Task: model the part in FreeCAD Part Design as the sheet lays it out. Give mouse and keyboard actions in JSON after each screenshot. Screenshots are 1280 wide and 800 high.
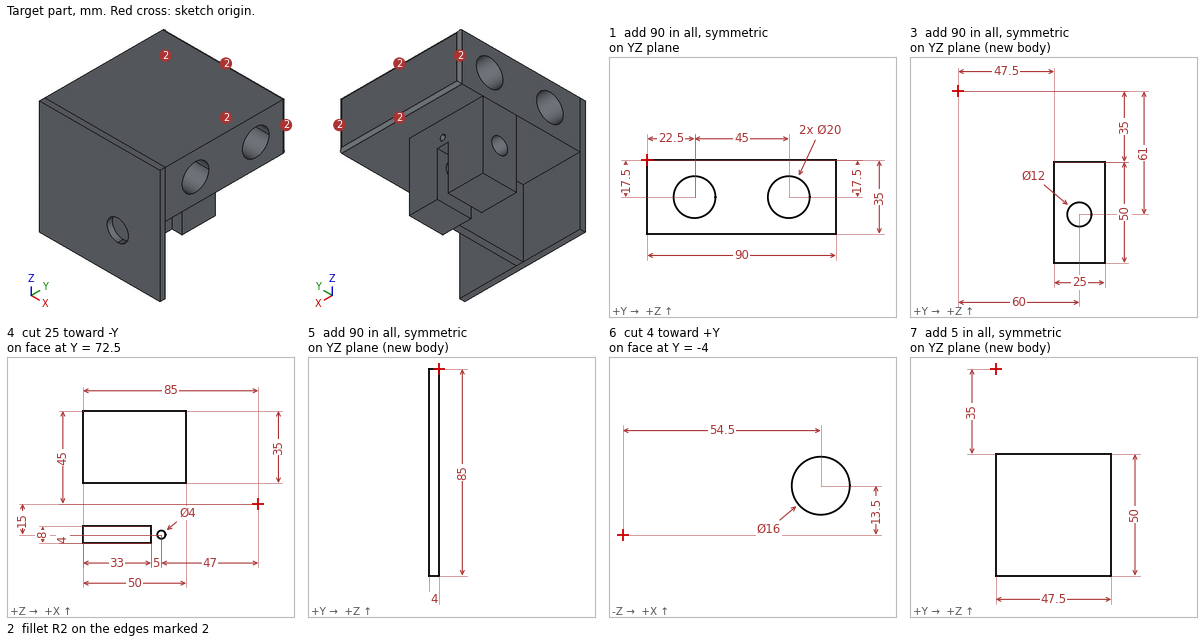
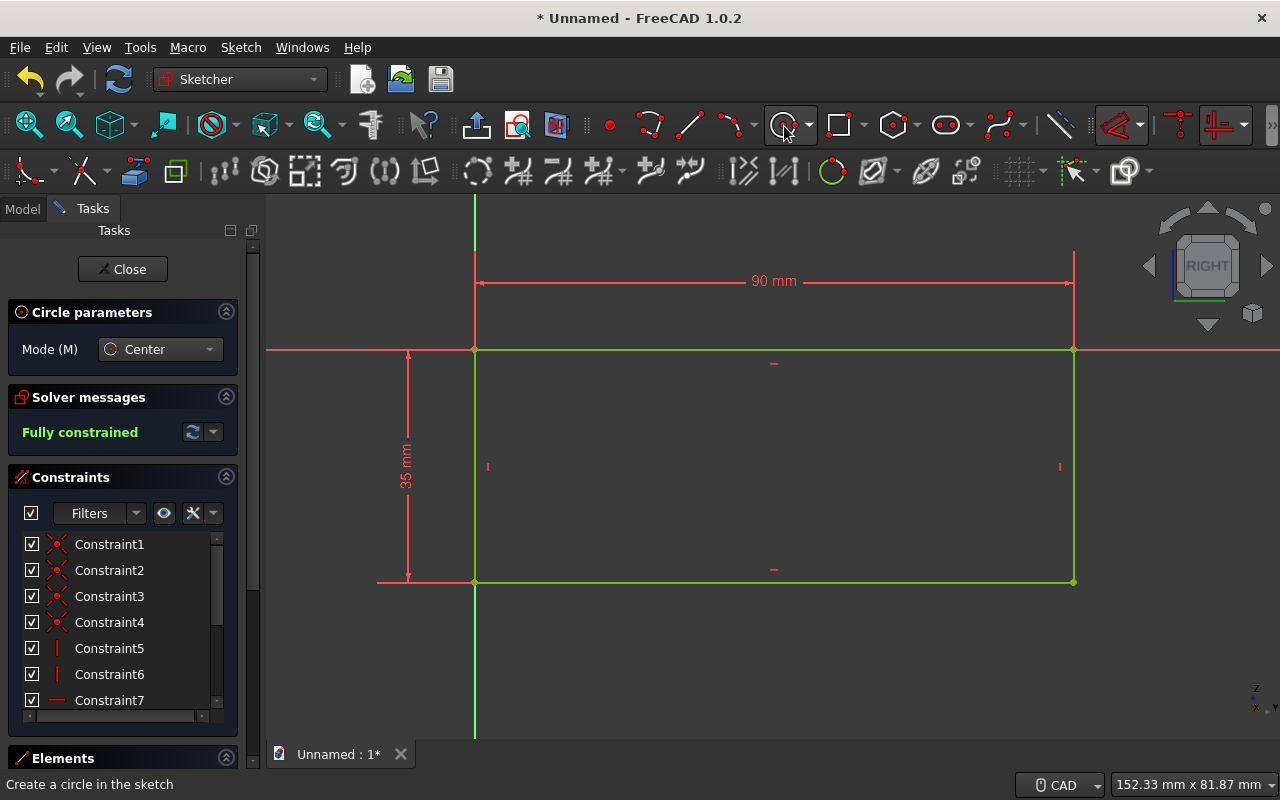
{"action": "left_click", "coordinate": [625, 466]}
{"action": "mouse_move", "coordinate": [672, 419]}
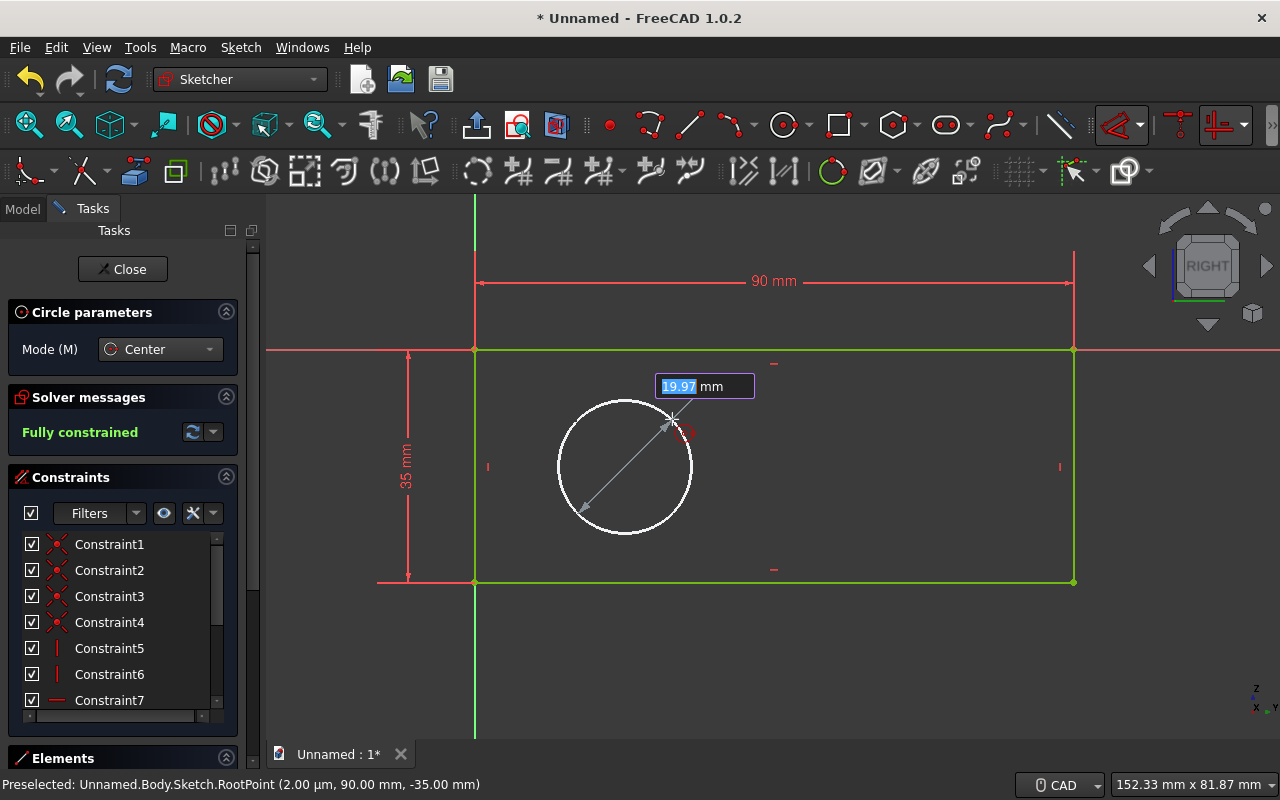
{"action": "type", "text": "20"}
{"action": "key", "text": "Return"}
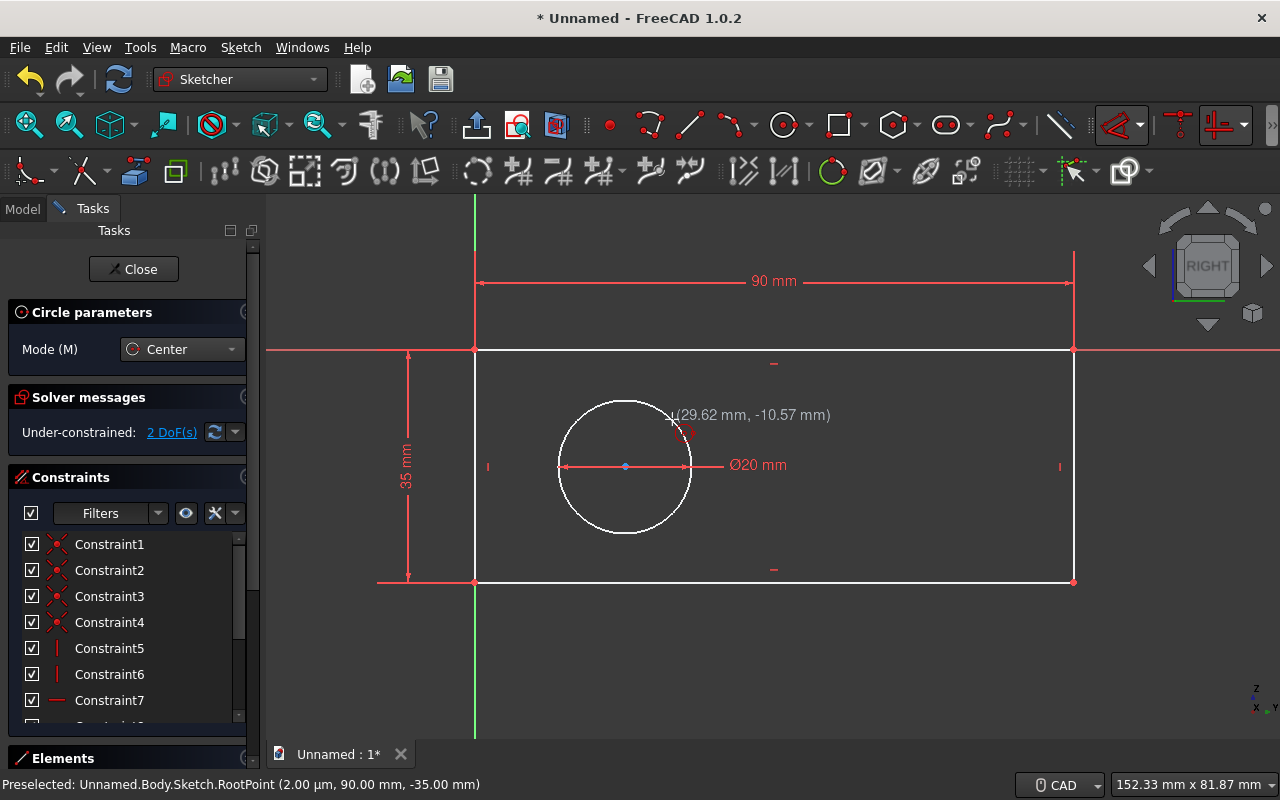
{"action": "left_click", "coordinate": [924, 466]}
{"action": "mouse_move", "coordinate": [971, 419]}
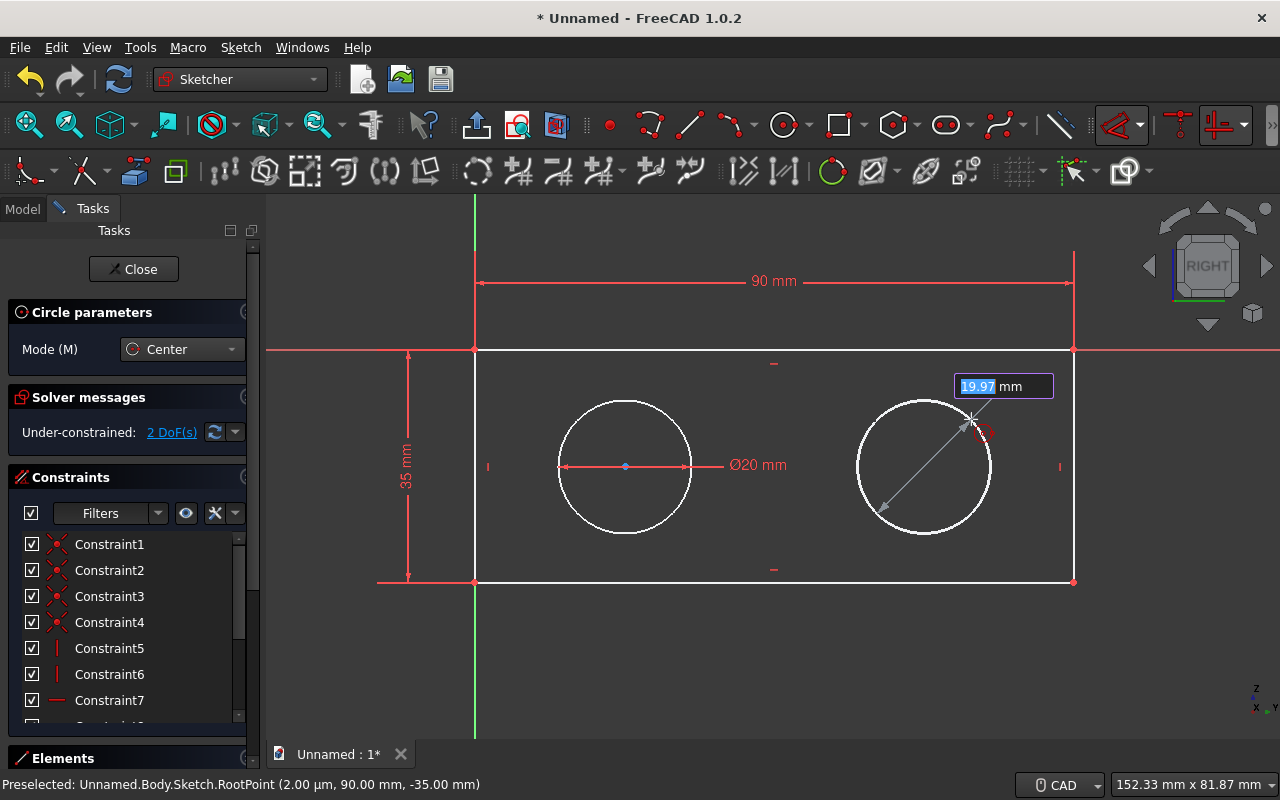
{"action": "type", "text": "20"}
{"action": "key", "text": "Return"}
{"action": "key", "text": "Escape"}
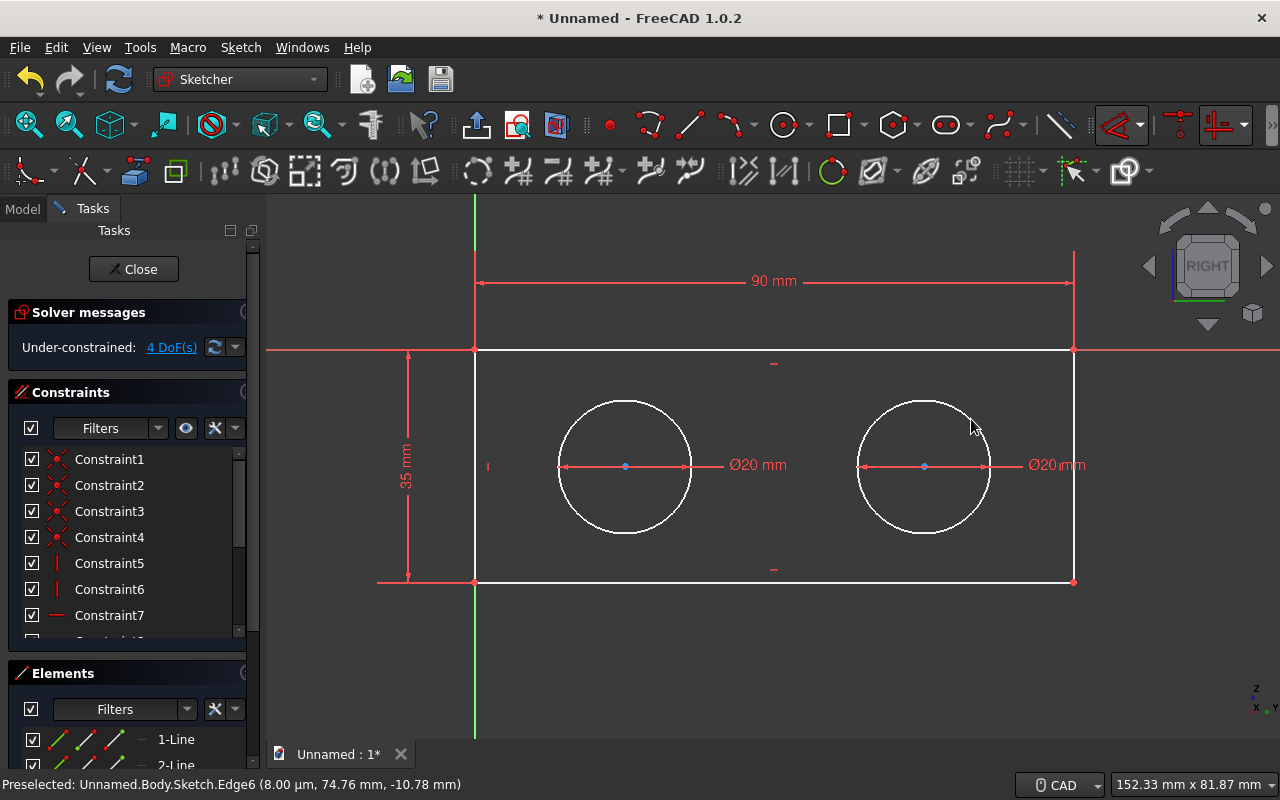
{"action": "left_click", "coordinate": [1116, 126]}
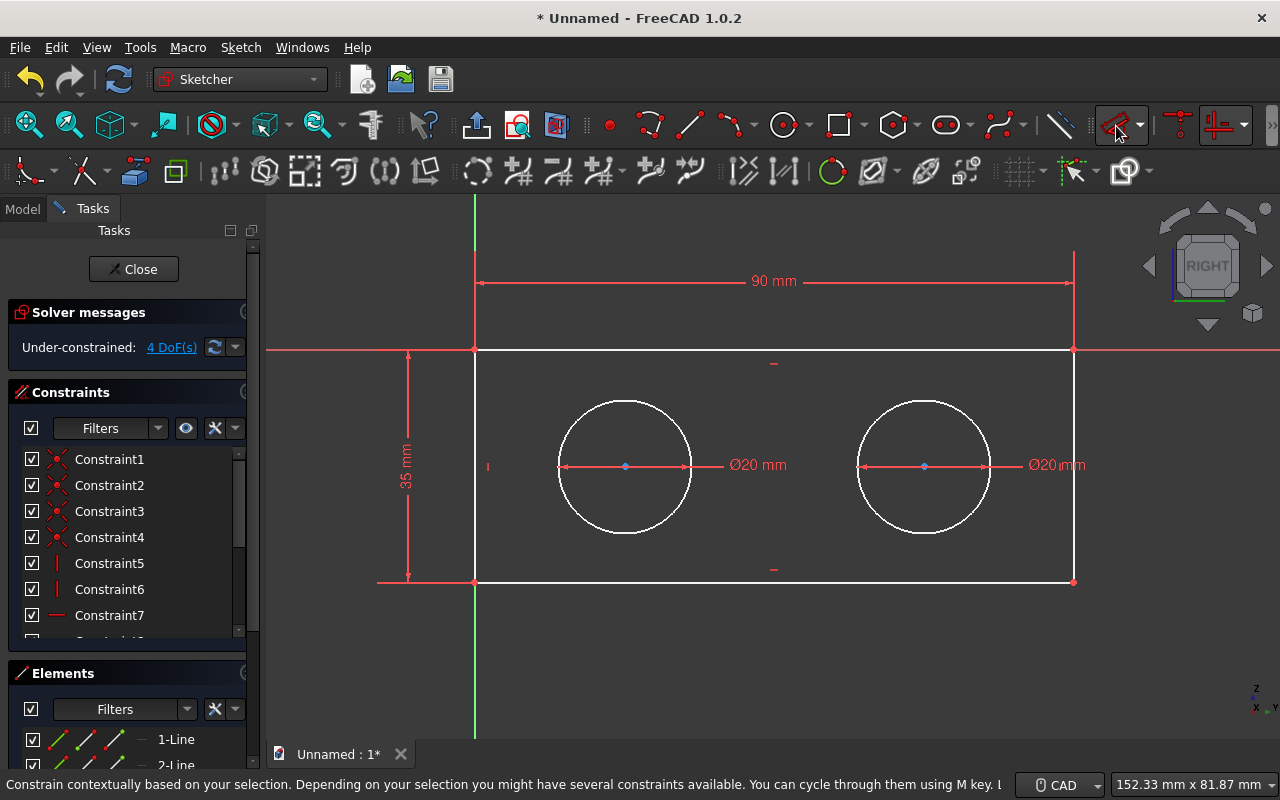
{"action": "left_click", "coordinate": [625, 467]}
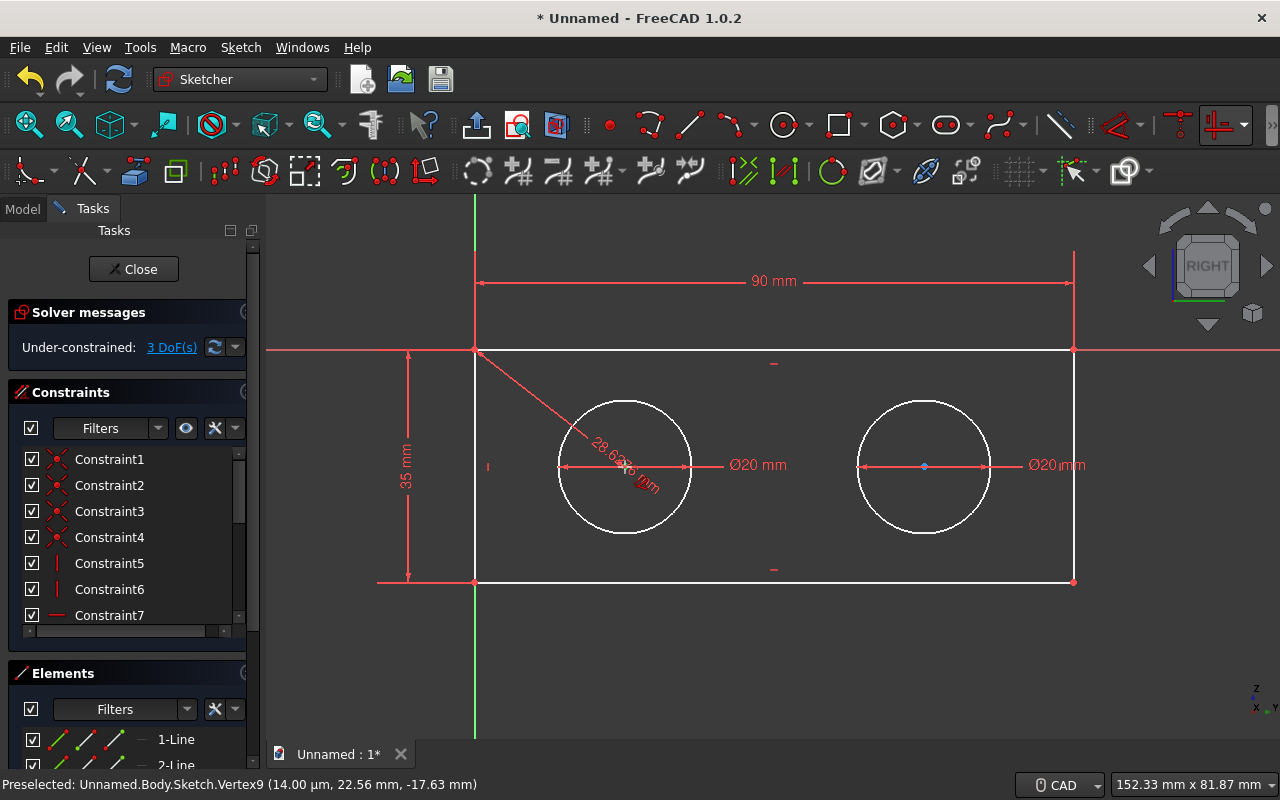
{"action": "left_click", "coordinate": [924, 467]}
{"action": "left_click", "coordinate": [774, 501]}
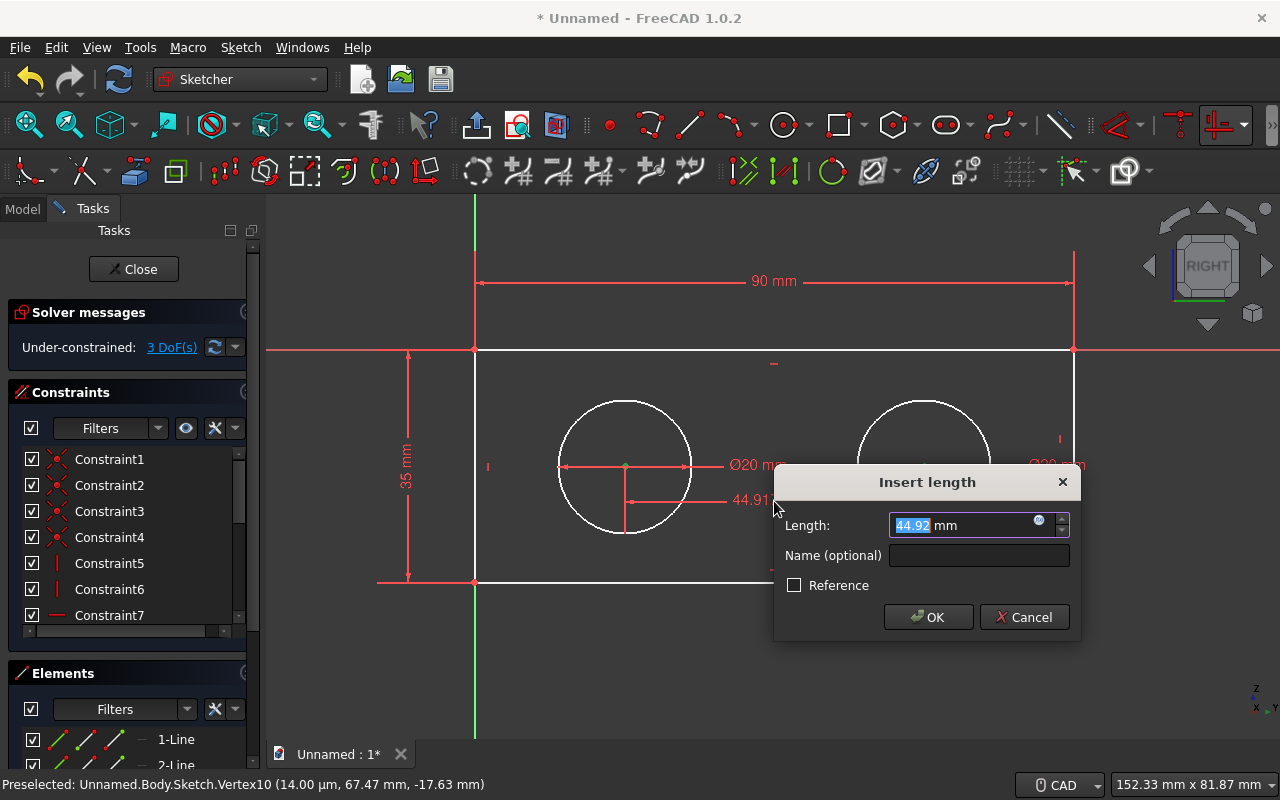
{"action": "type", "text": "45"}
{"action": "key", "text": "Return"}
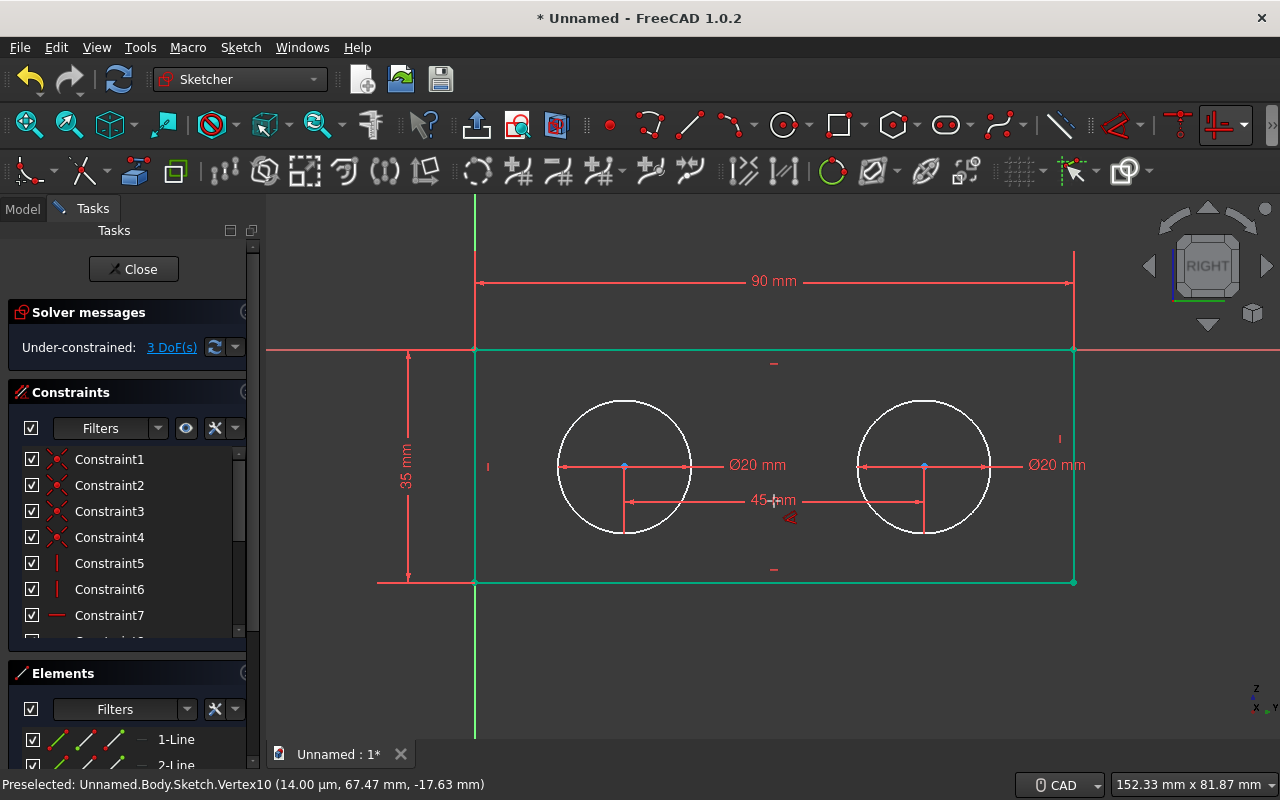
{"action": "left_click", "coordinate": [624, 467]}
{"action": "left_click", "coordinate": [550, 316]}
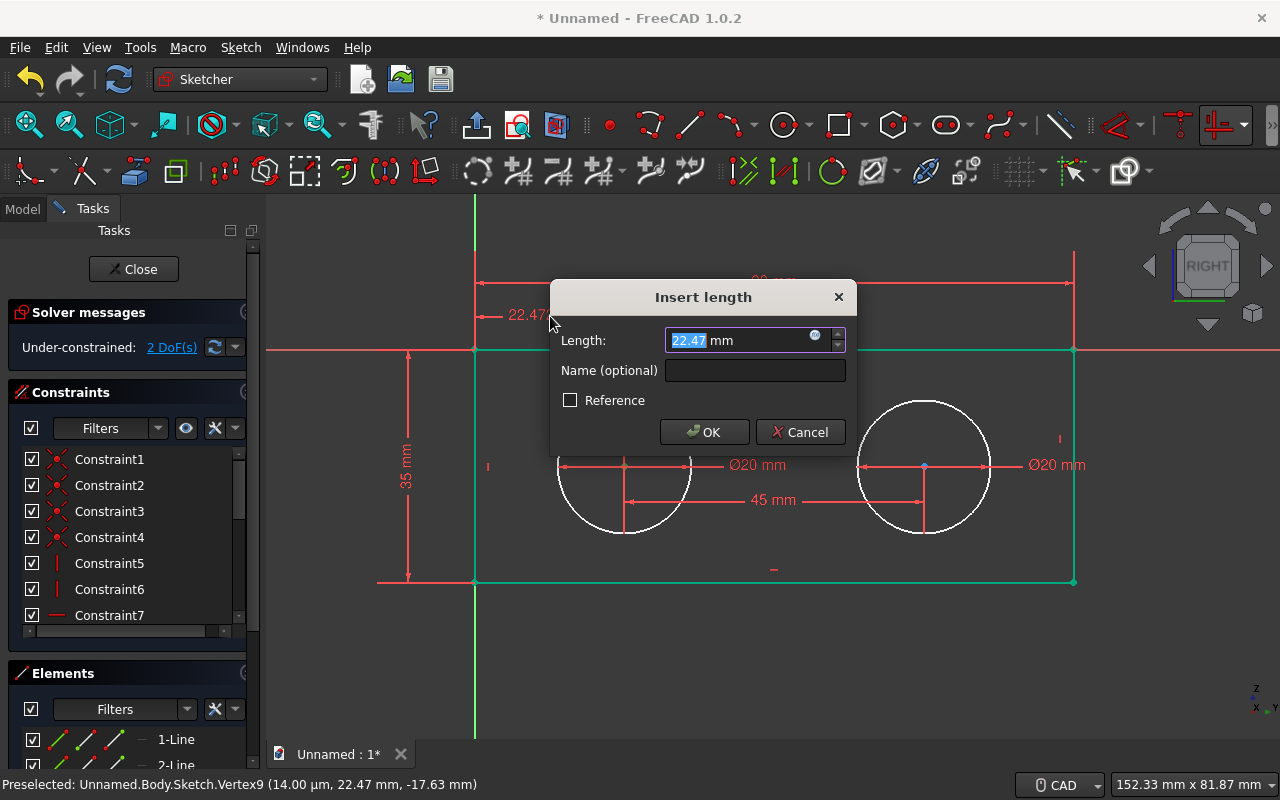
{"action": "type", "text": "22.5"}
{"action": "key", "text": "Return"}